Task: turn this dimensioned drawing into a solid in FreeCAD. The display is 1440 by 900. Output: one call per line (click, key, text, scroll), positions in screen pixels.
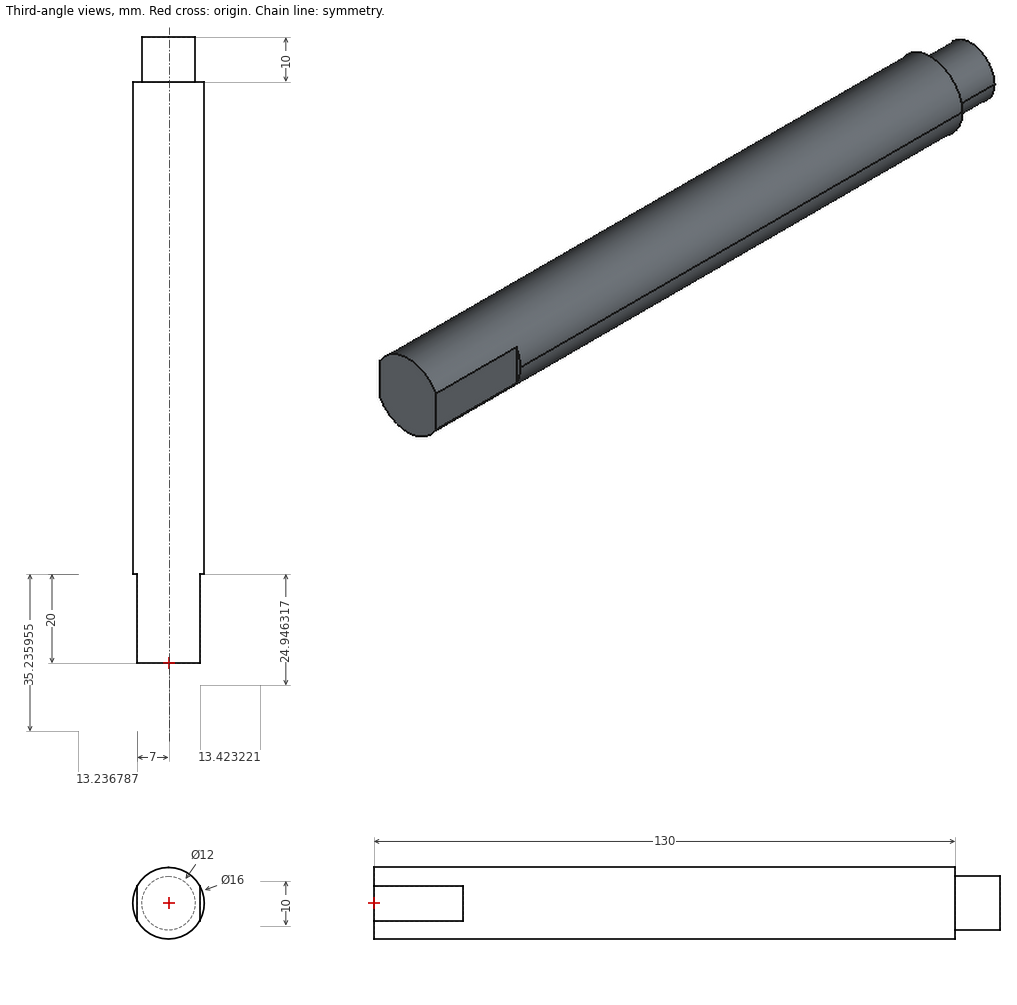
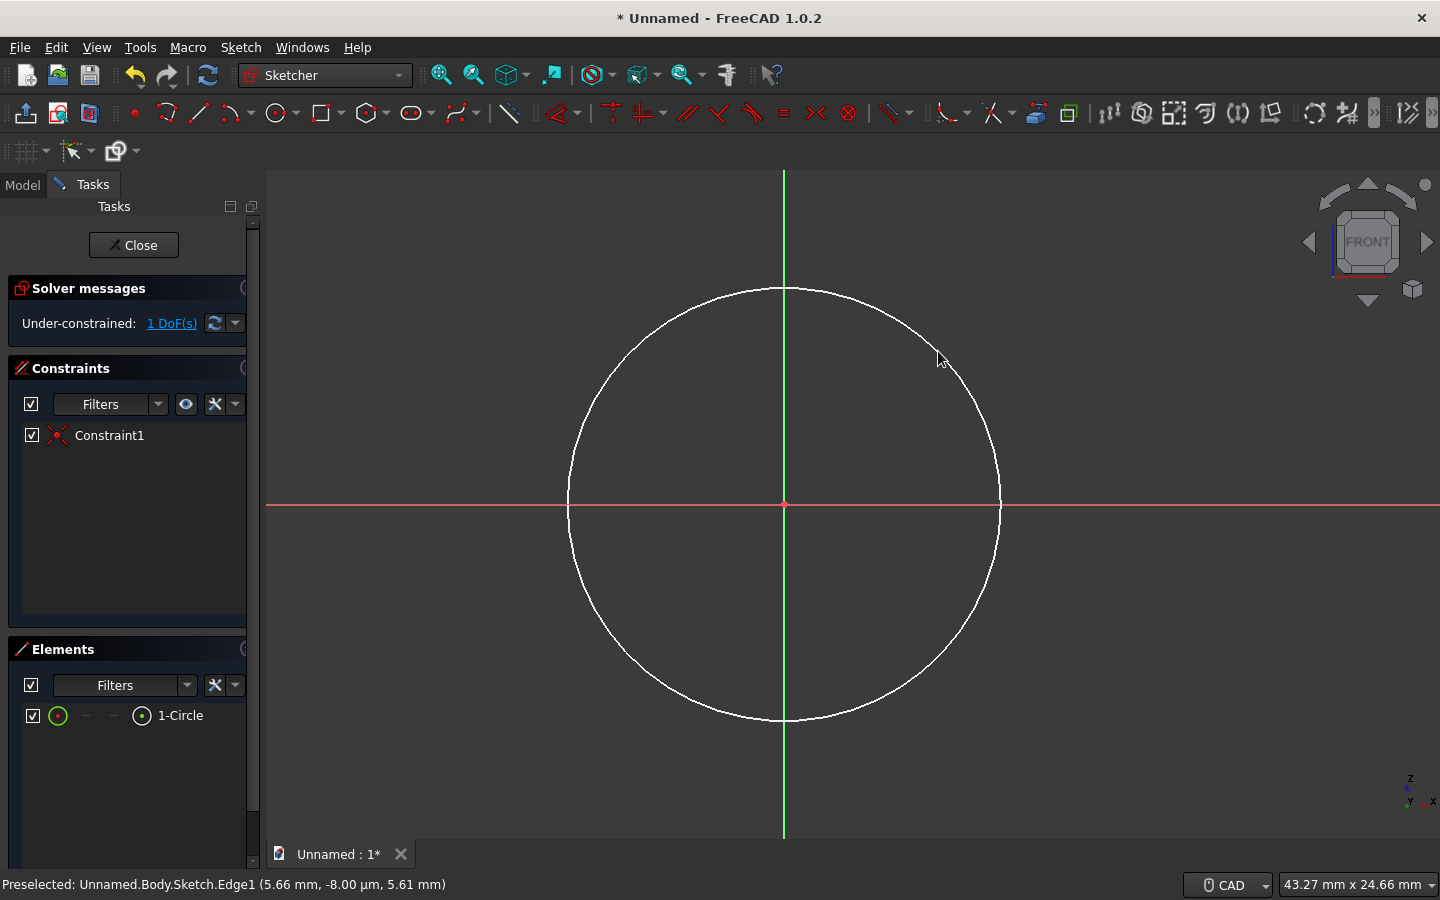
click(556, 114)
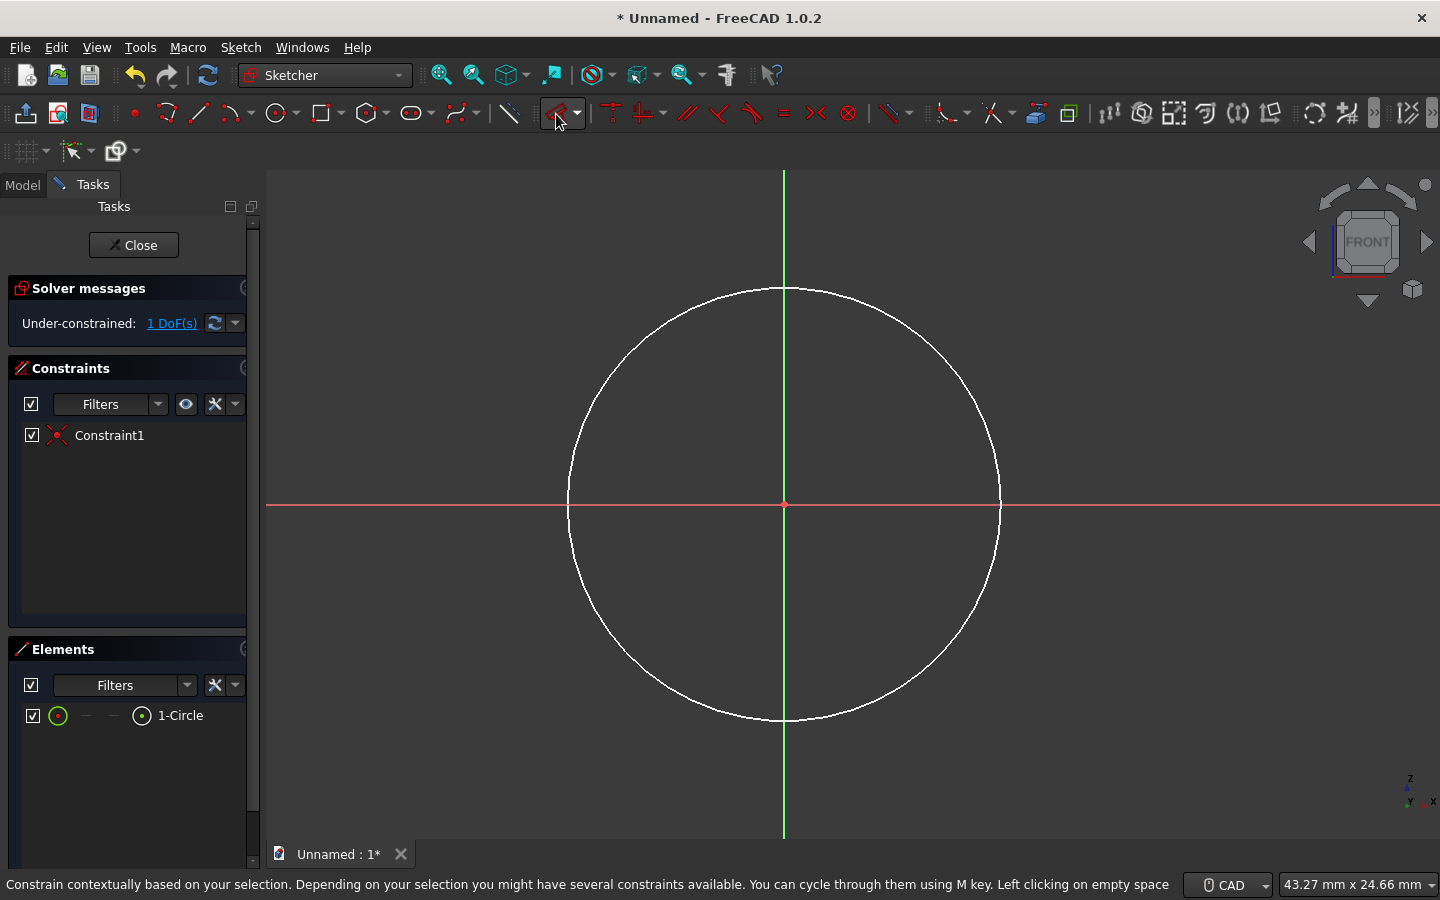
click(937, 351)
click(960, 328)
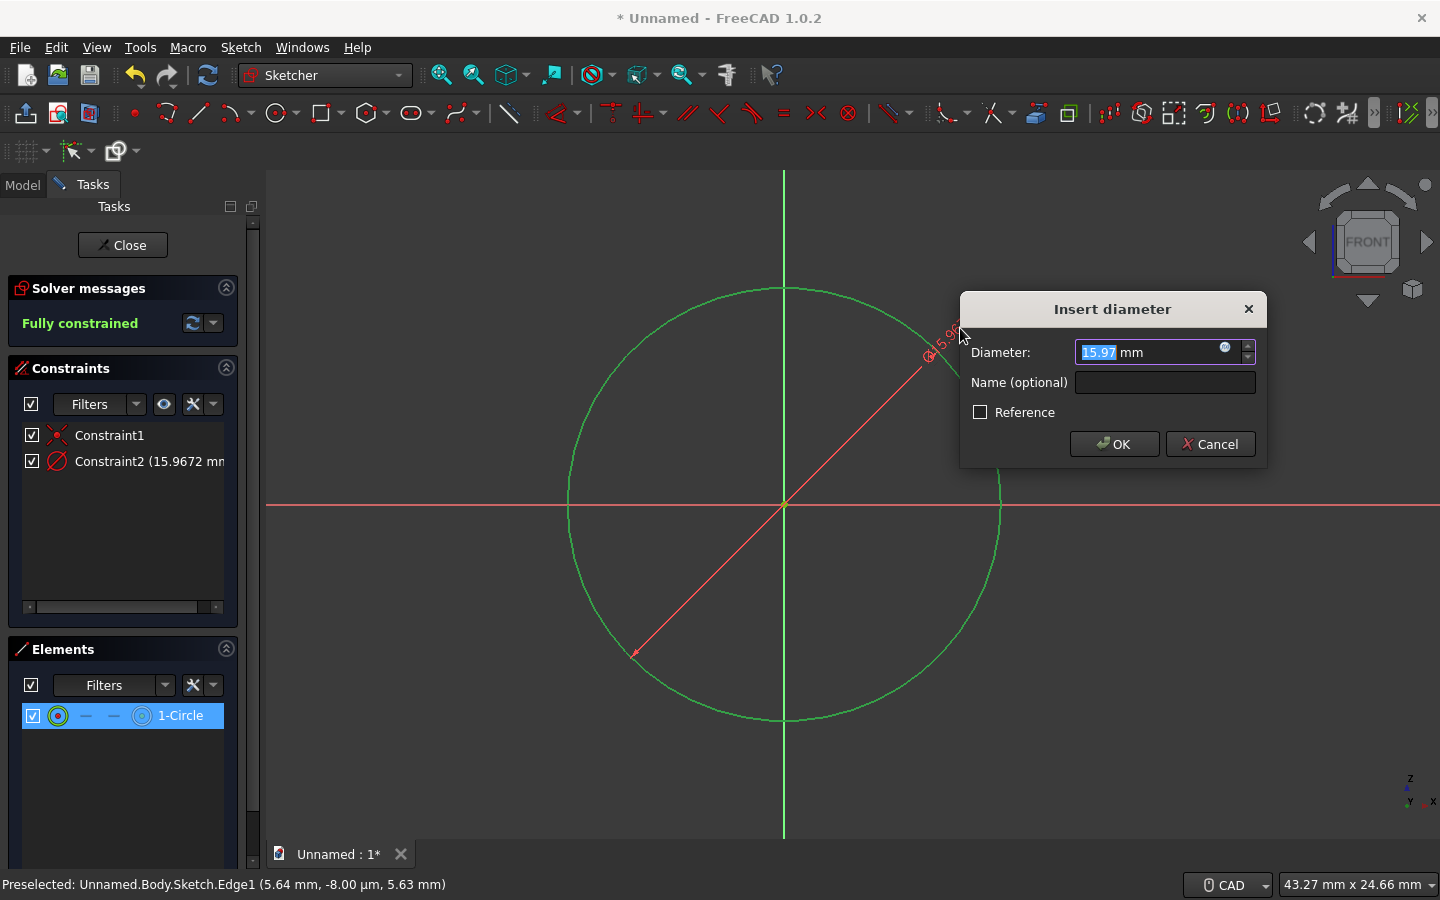
text(16)
key(Return)
key(Escape)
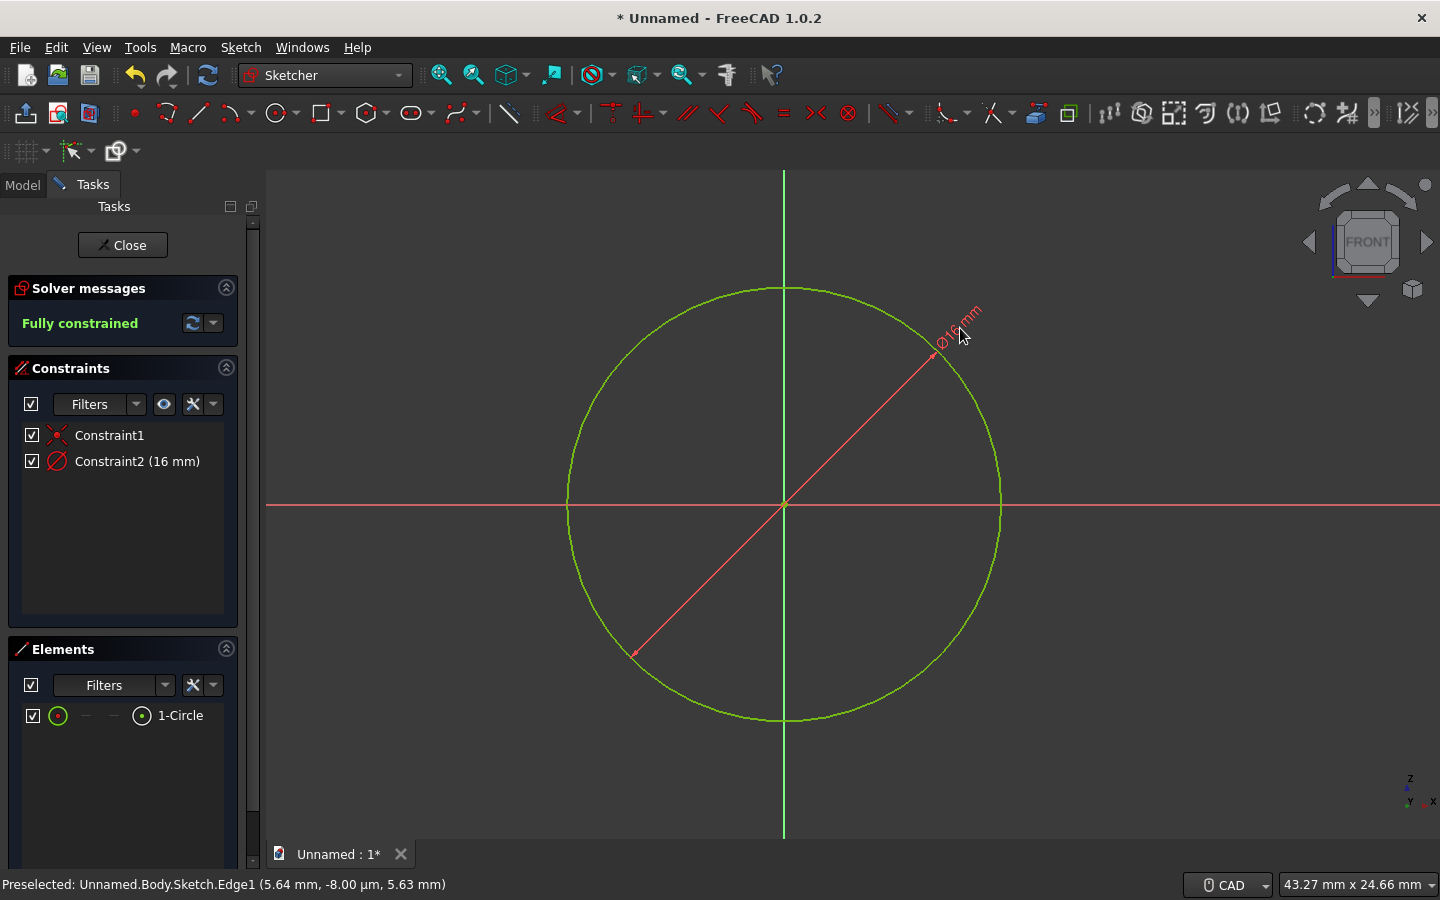
click(123, 245)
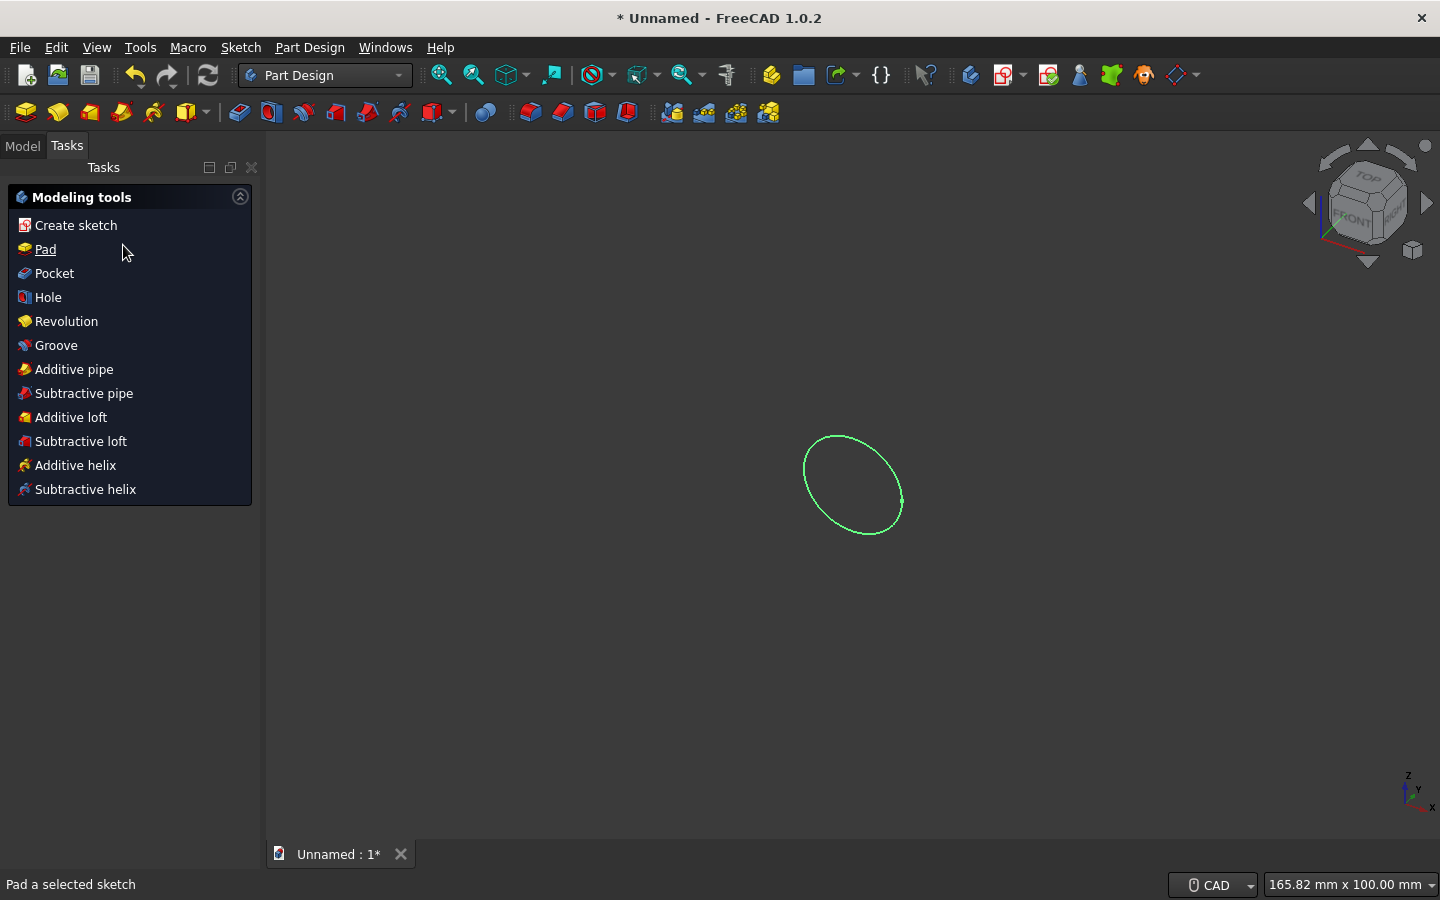
click(26, 112)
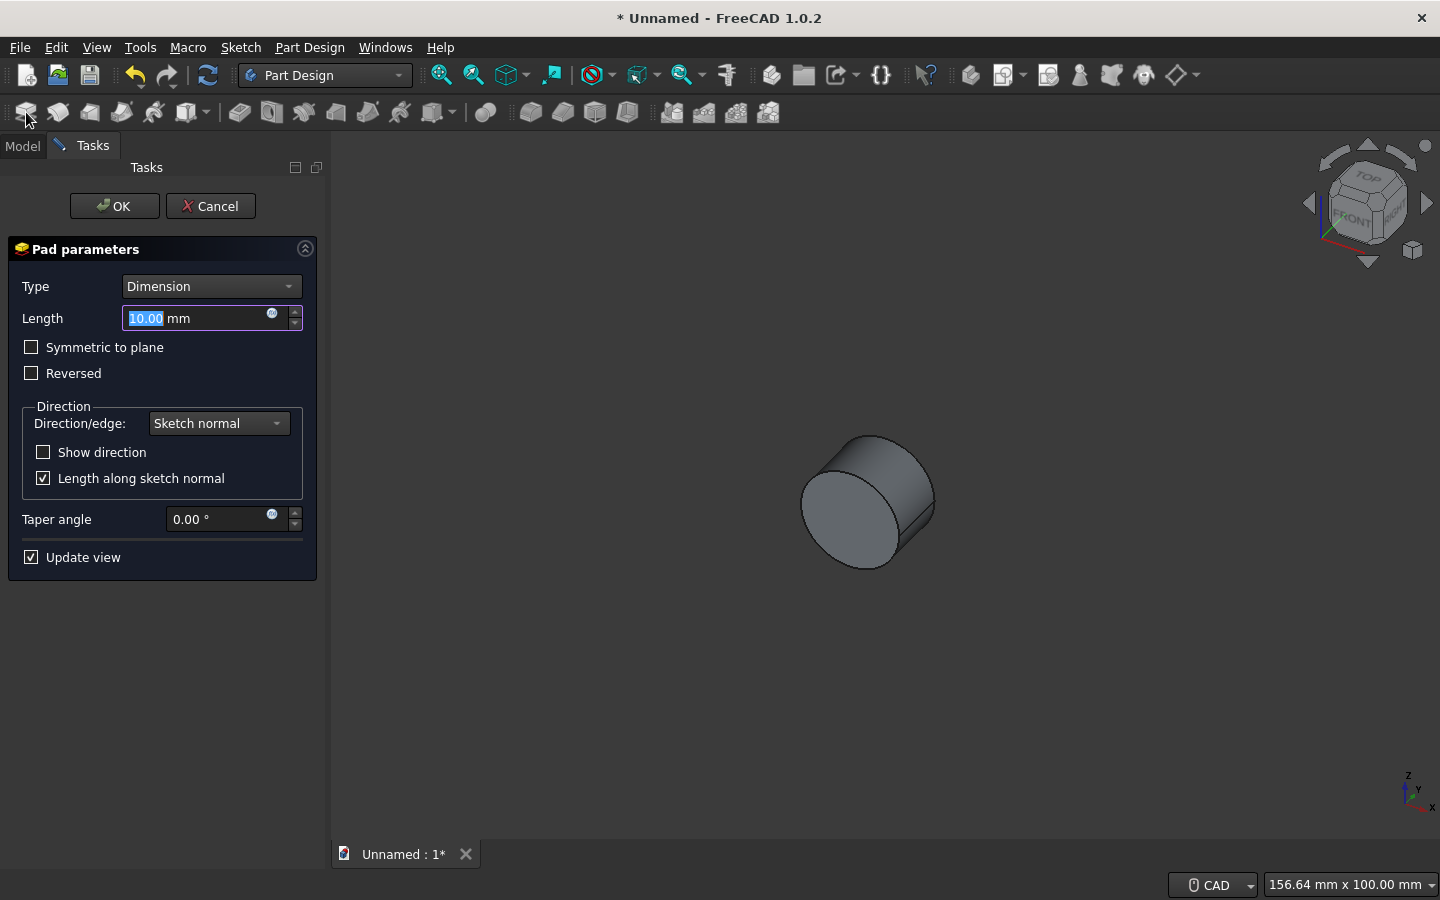
text(130)
key(Tab)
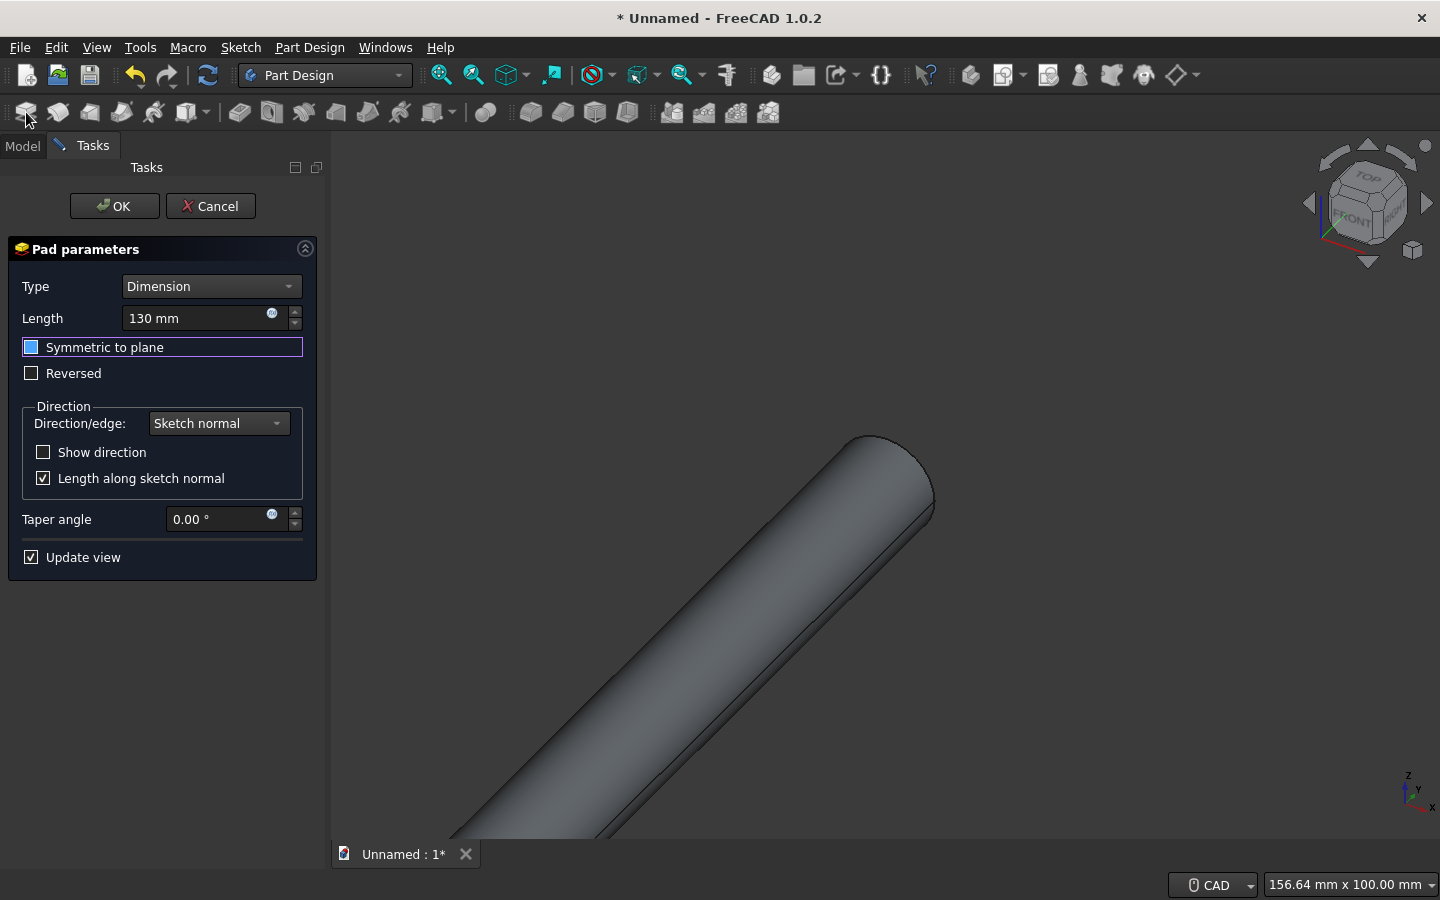
click(30, 373)